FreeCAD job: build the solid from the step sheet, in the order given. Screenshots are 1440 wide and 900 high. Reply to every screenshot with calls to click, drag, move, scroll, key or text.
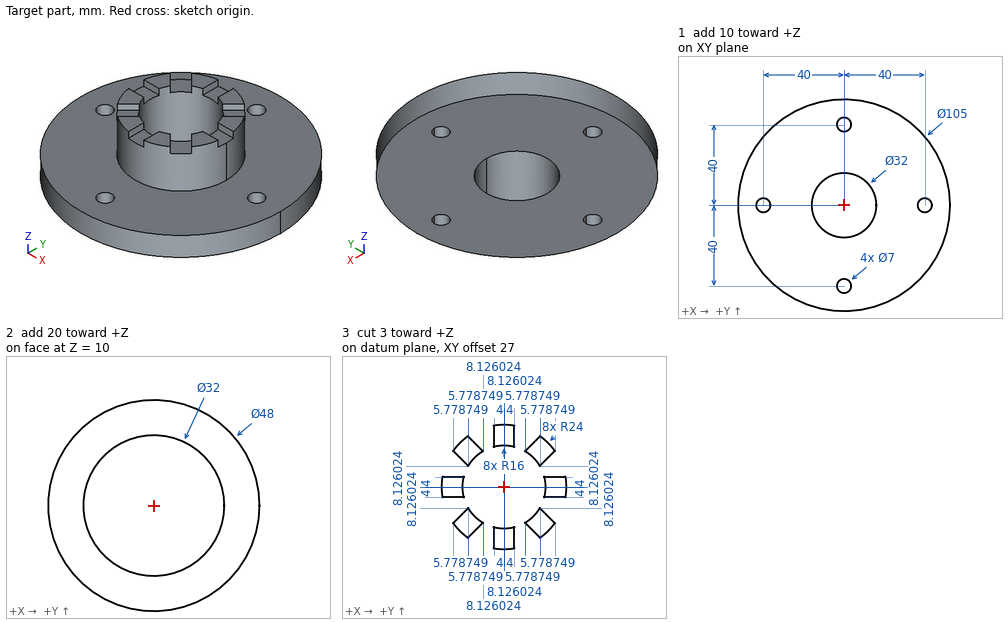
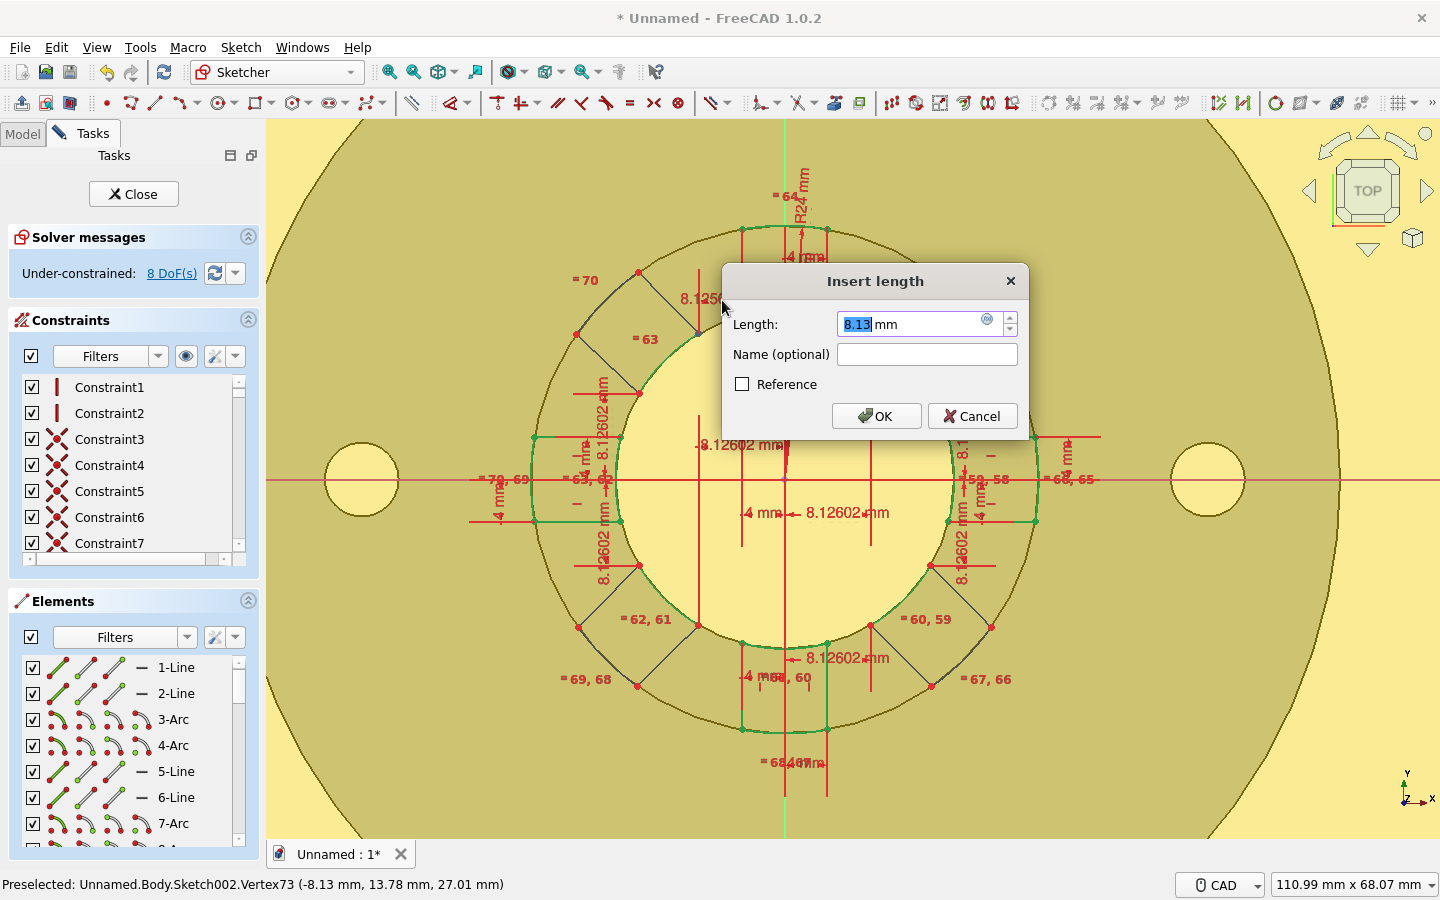
text(8.126024)
key(Return)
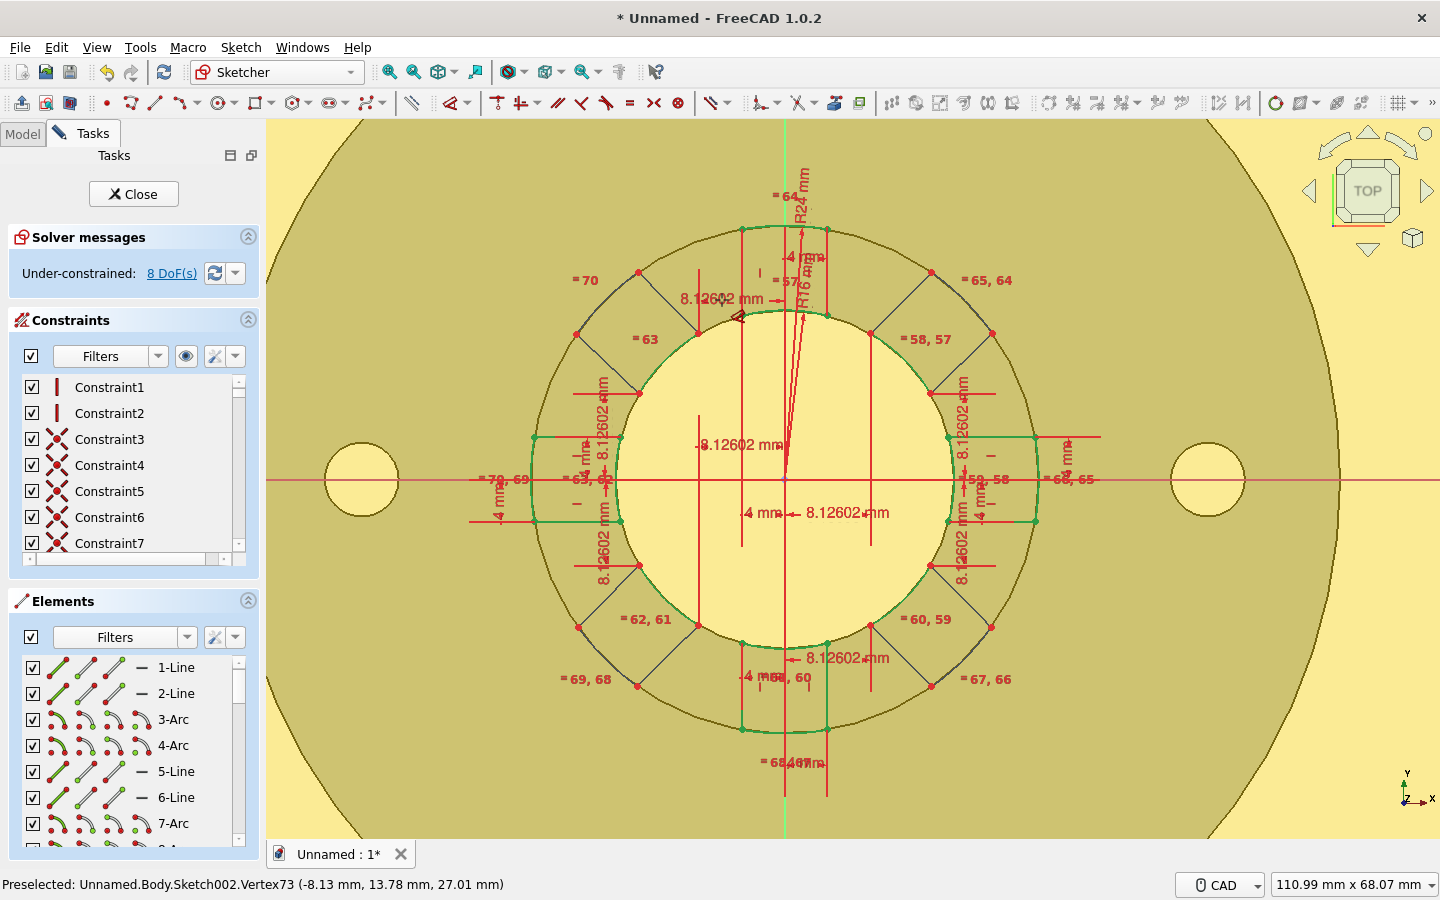
click(913, 291)
click(901, 239)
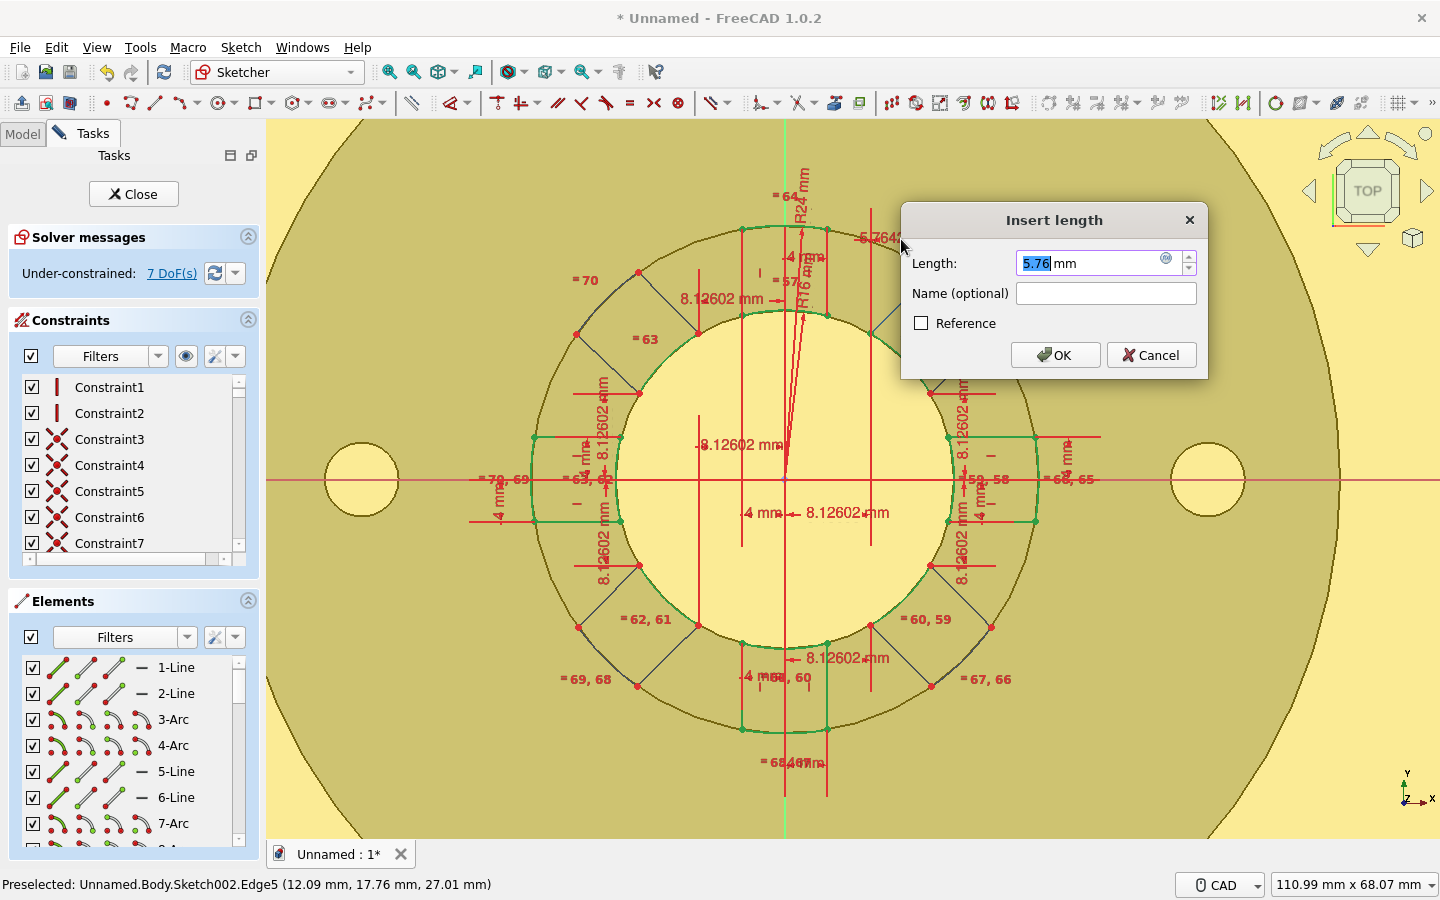
text(5.778749)
key(Return)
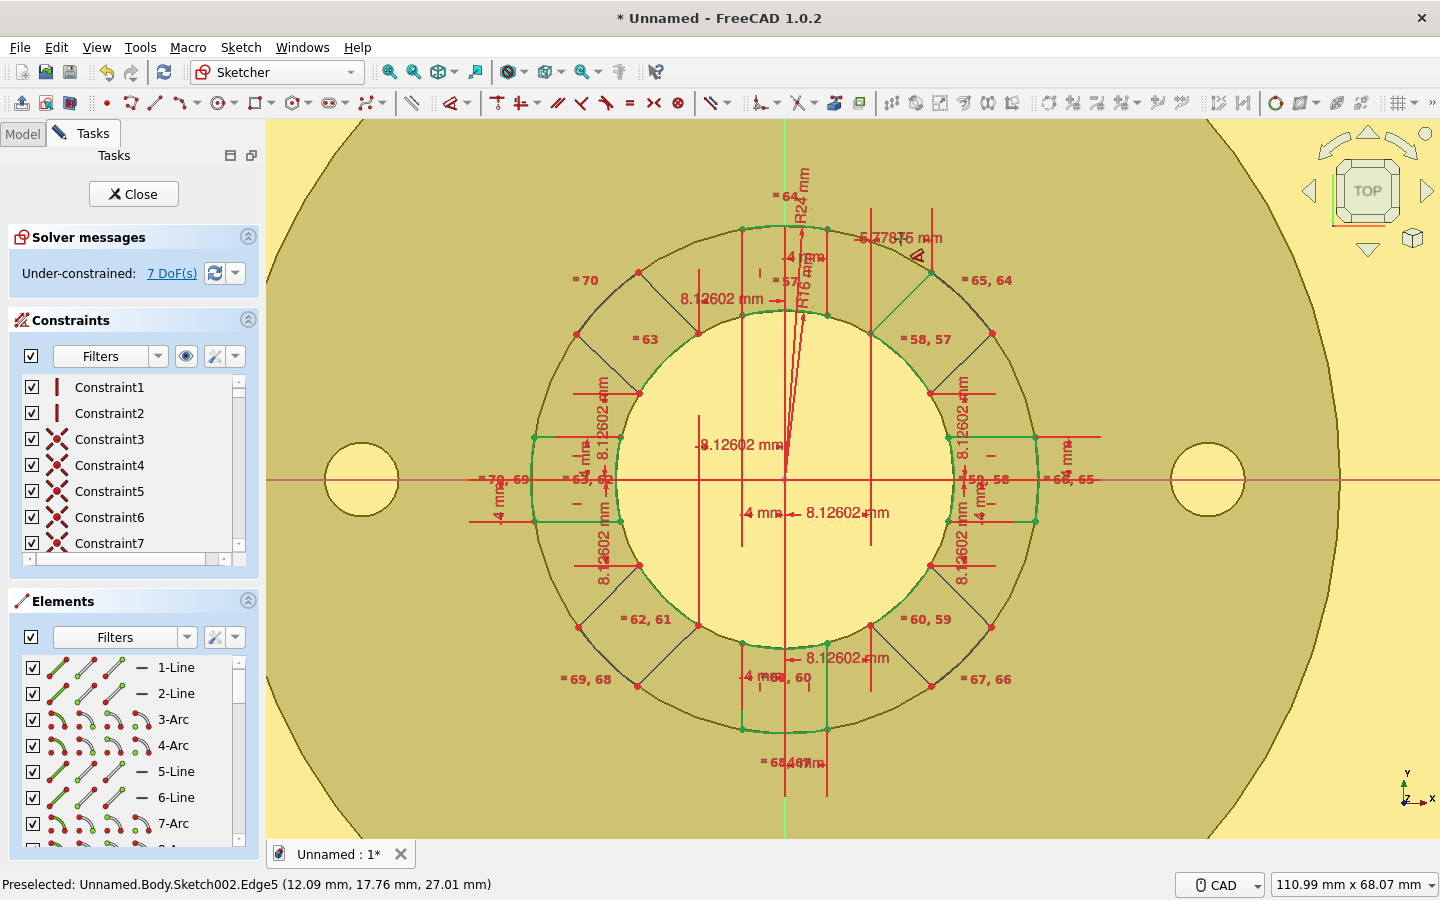
click(949, 376)
click(940, 299)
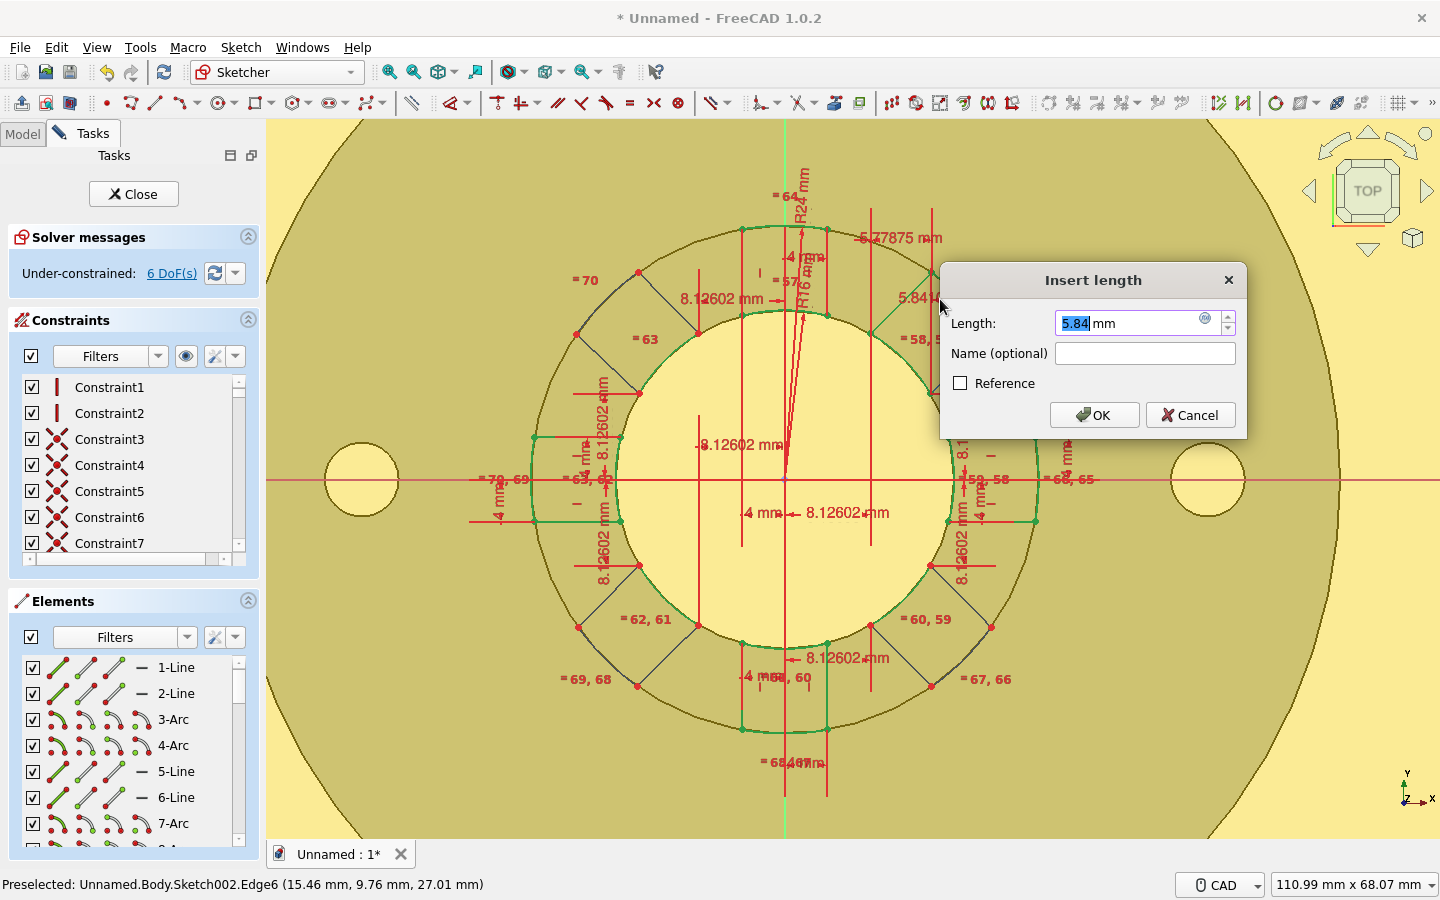
text(5.778749)
key(Return)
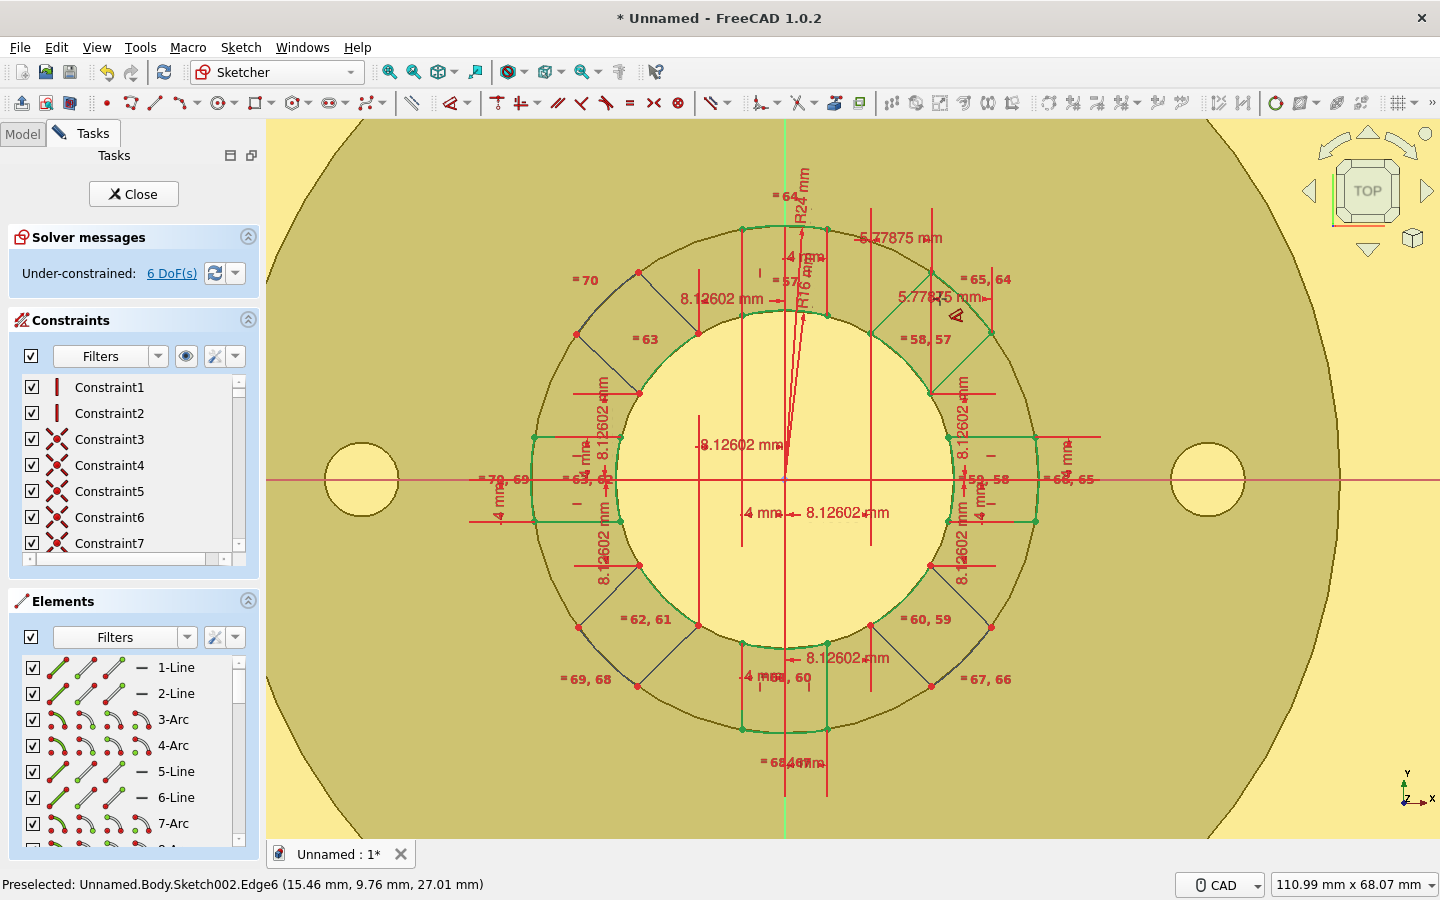
click(973, 609)
click(940, 661)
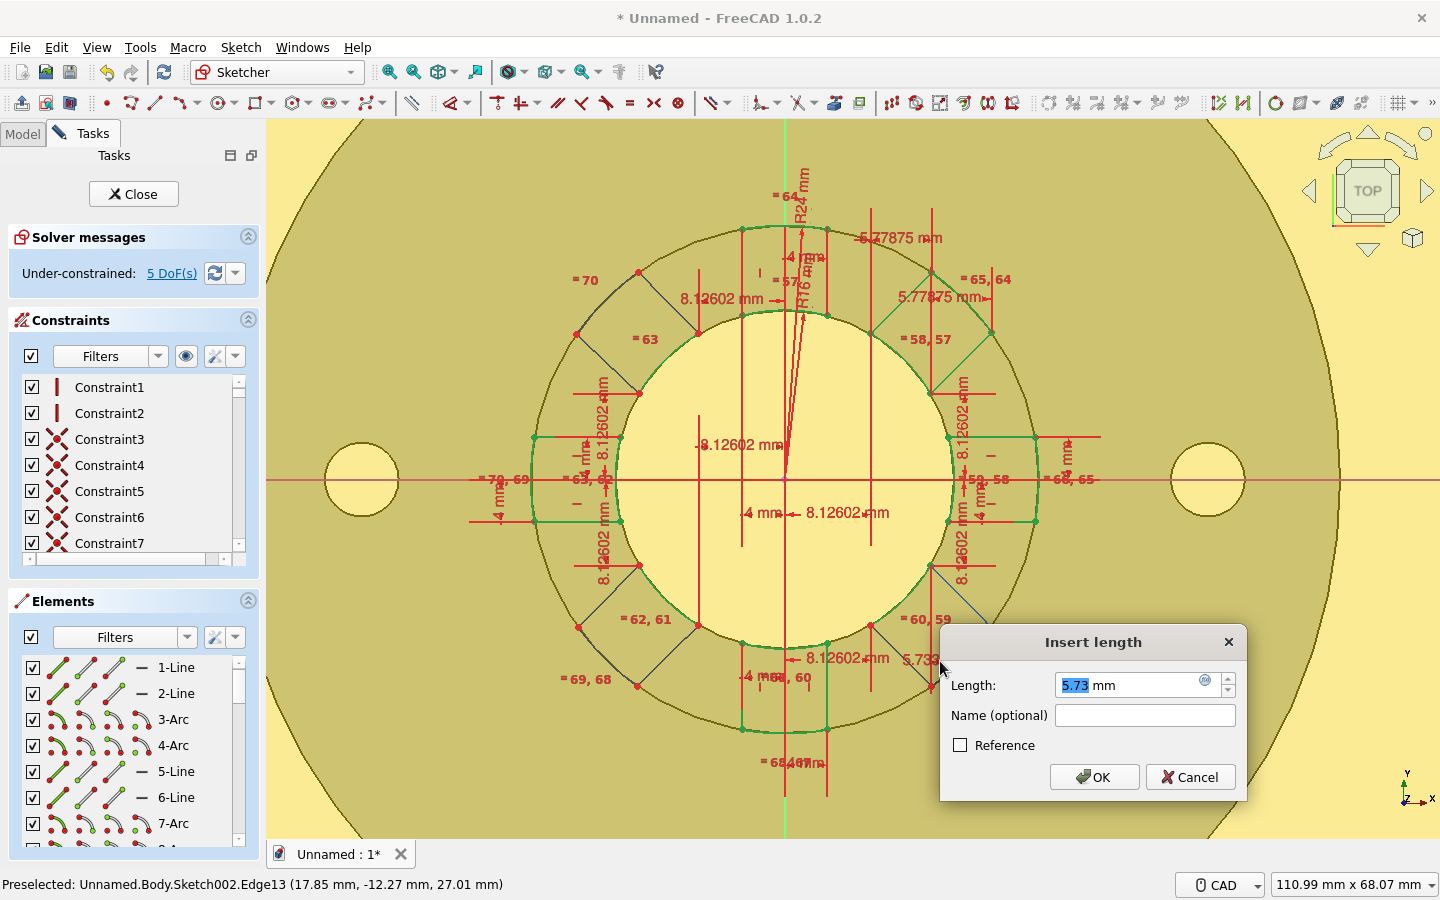
text(5.778749)
key(Return)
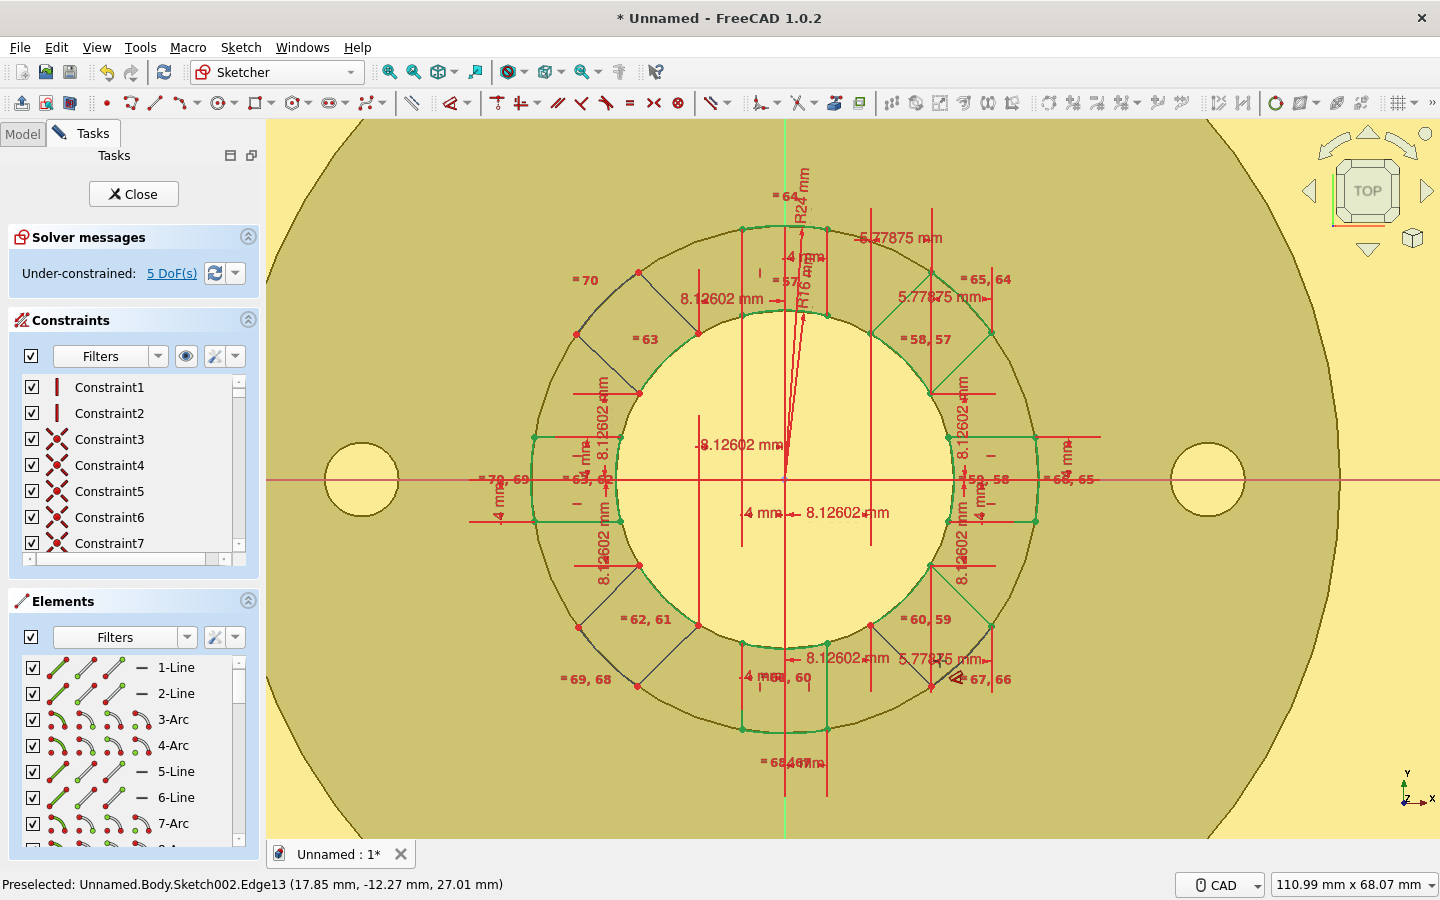
click(889, 644)
click(901, 721)